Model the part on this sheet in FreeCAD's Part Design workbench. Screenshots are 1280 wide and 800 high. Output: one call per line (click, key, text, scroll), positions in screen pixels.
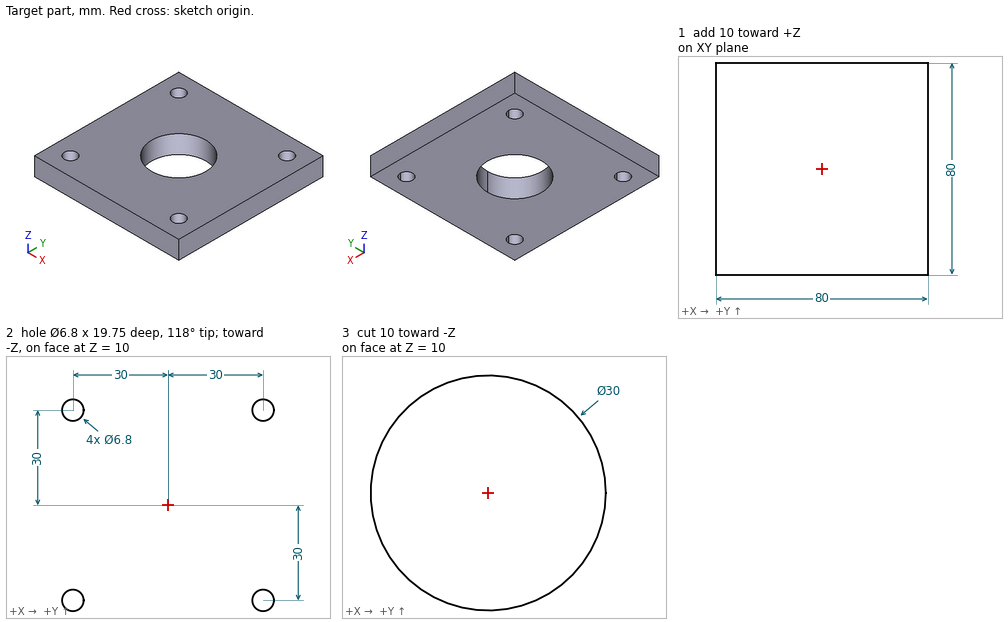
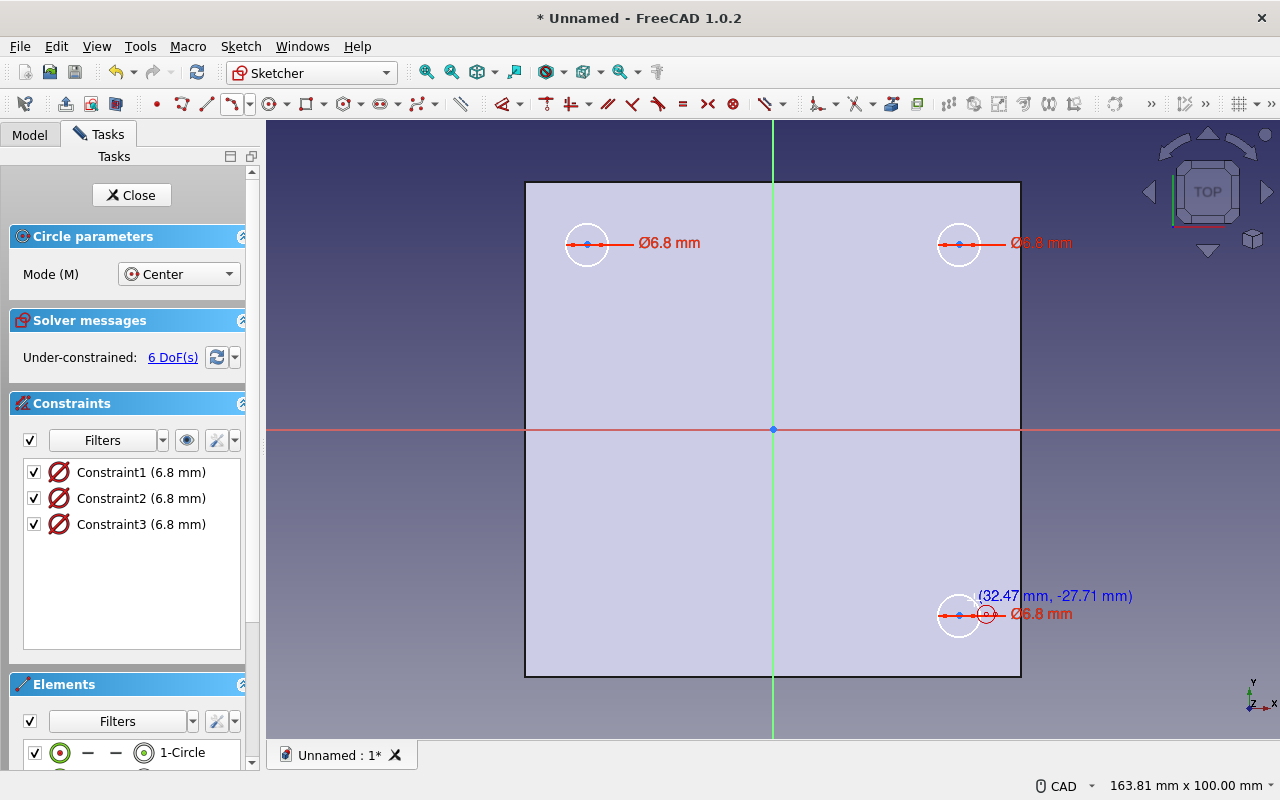
click(587, 615)
move(602, 600)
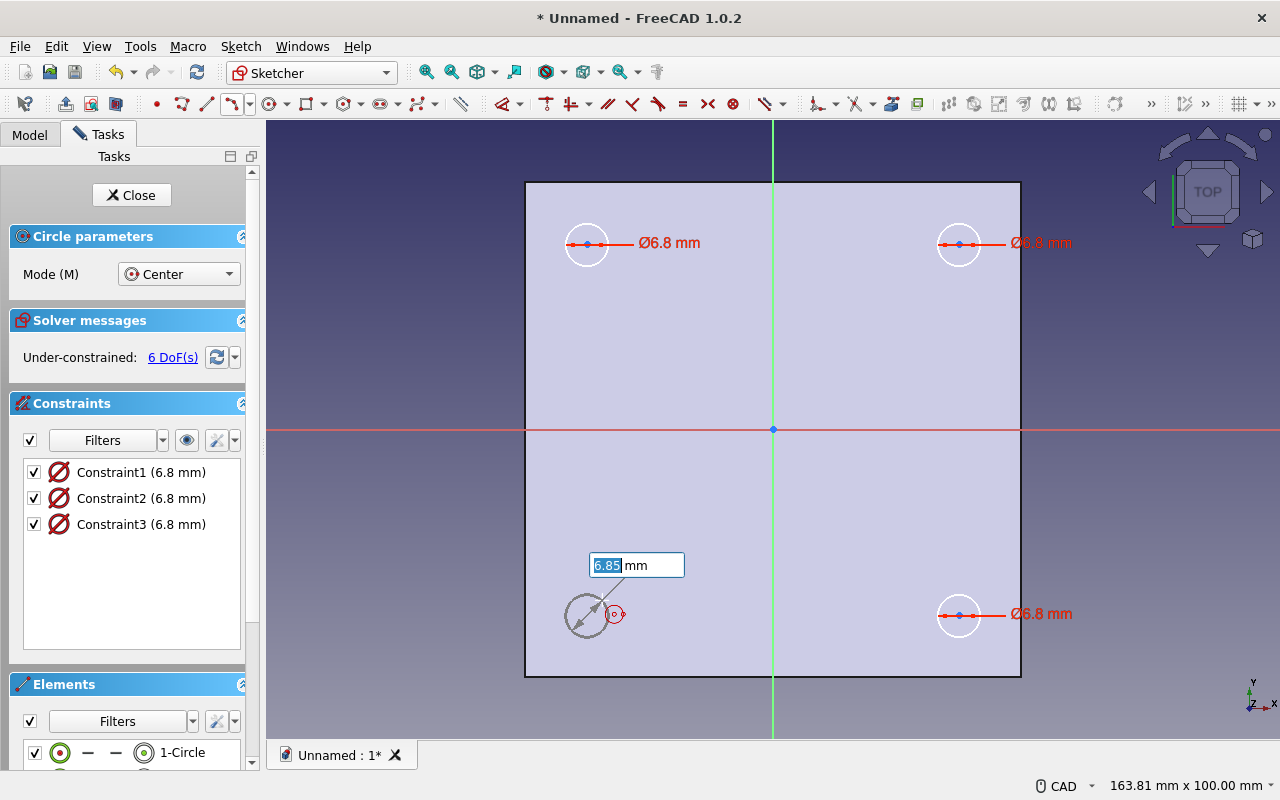
text(6.8)
key(Return)
key(Escape)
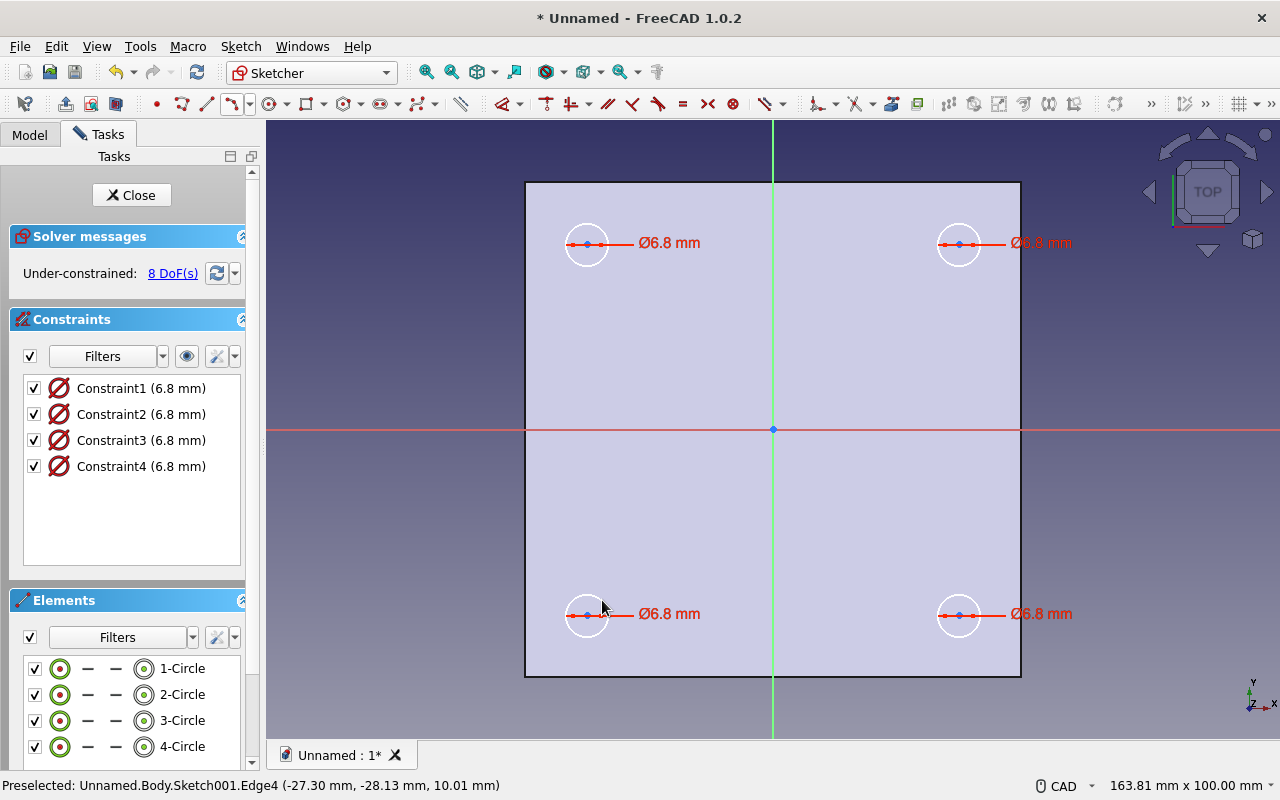
click(587, 245)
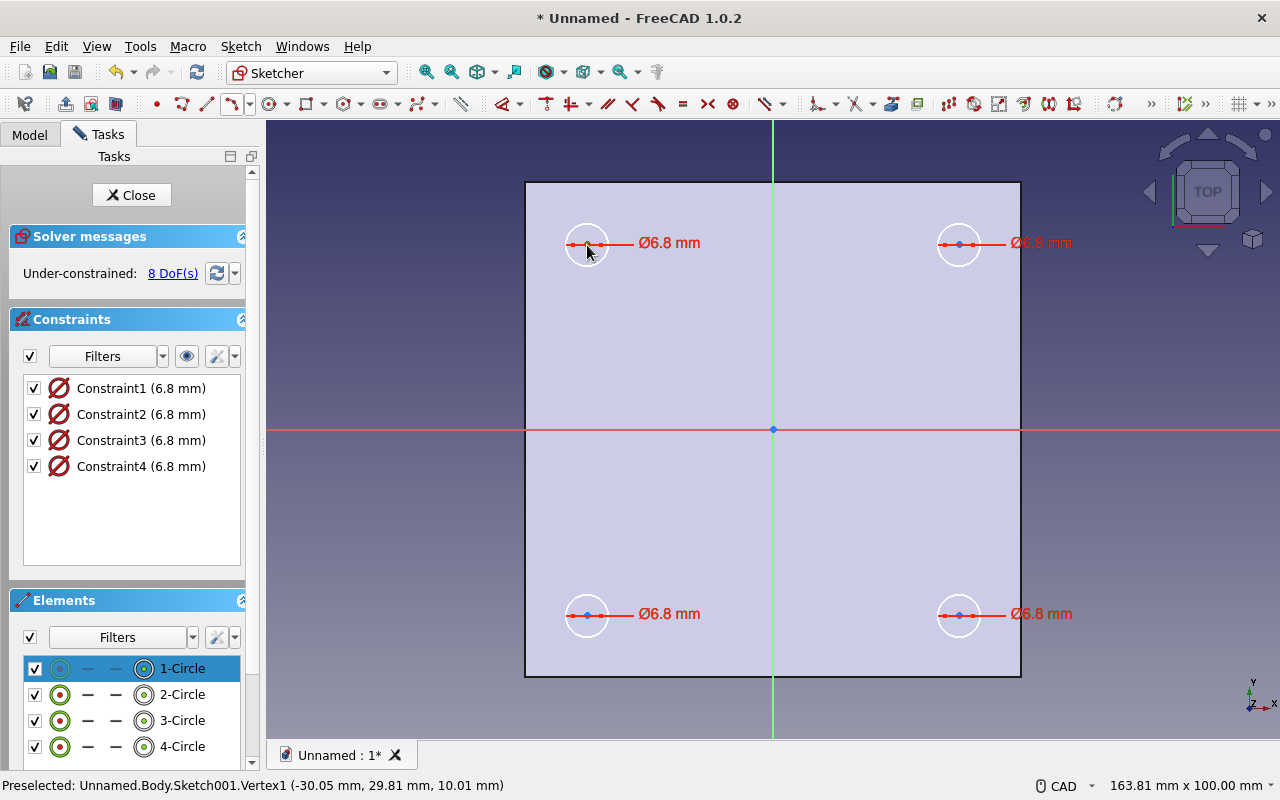
click(959, 245)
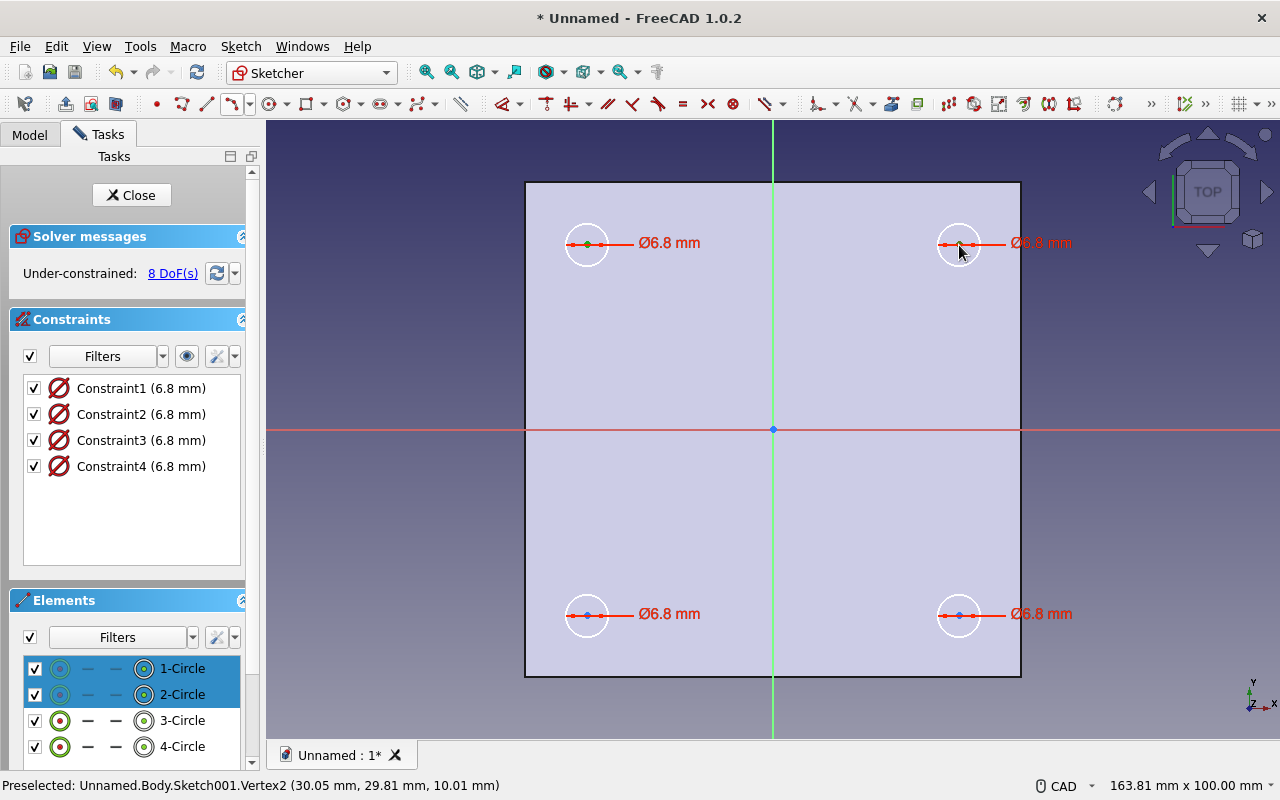
click(588, 104)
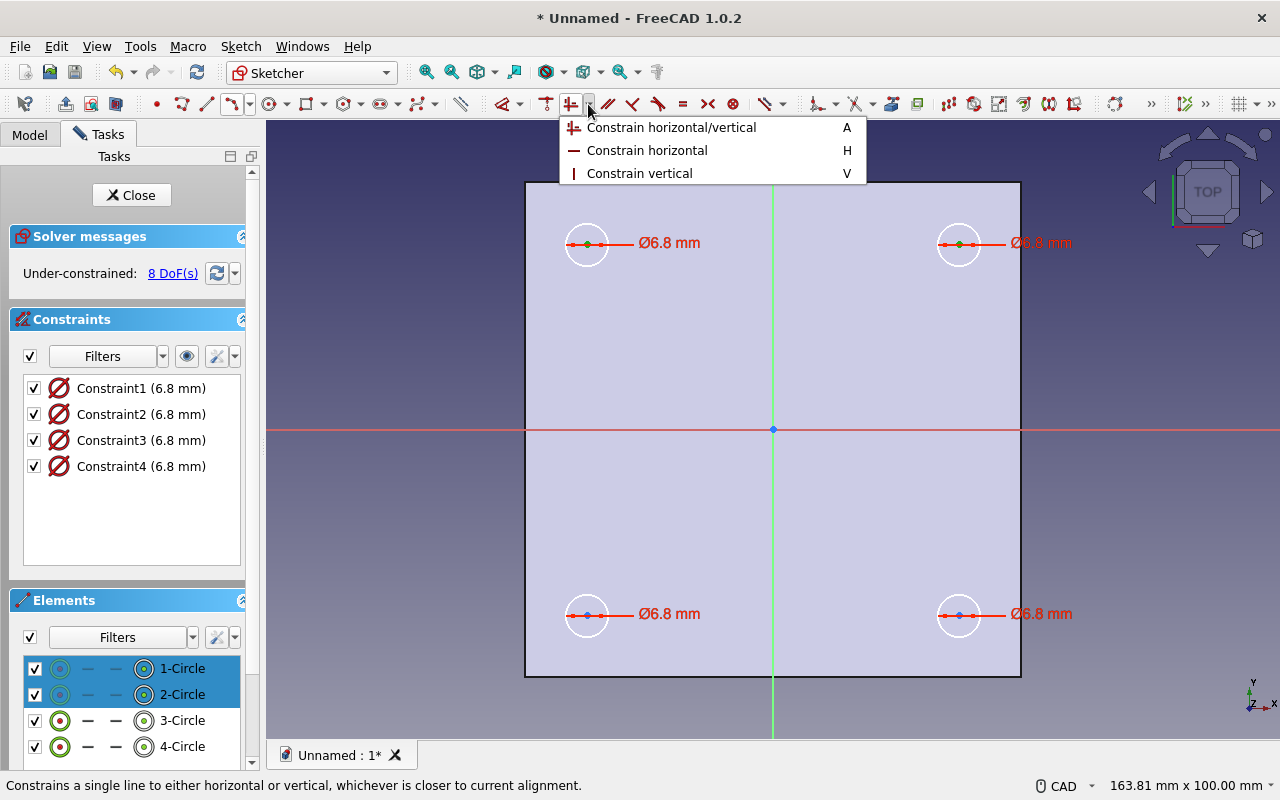
click(713, 150)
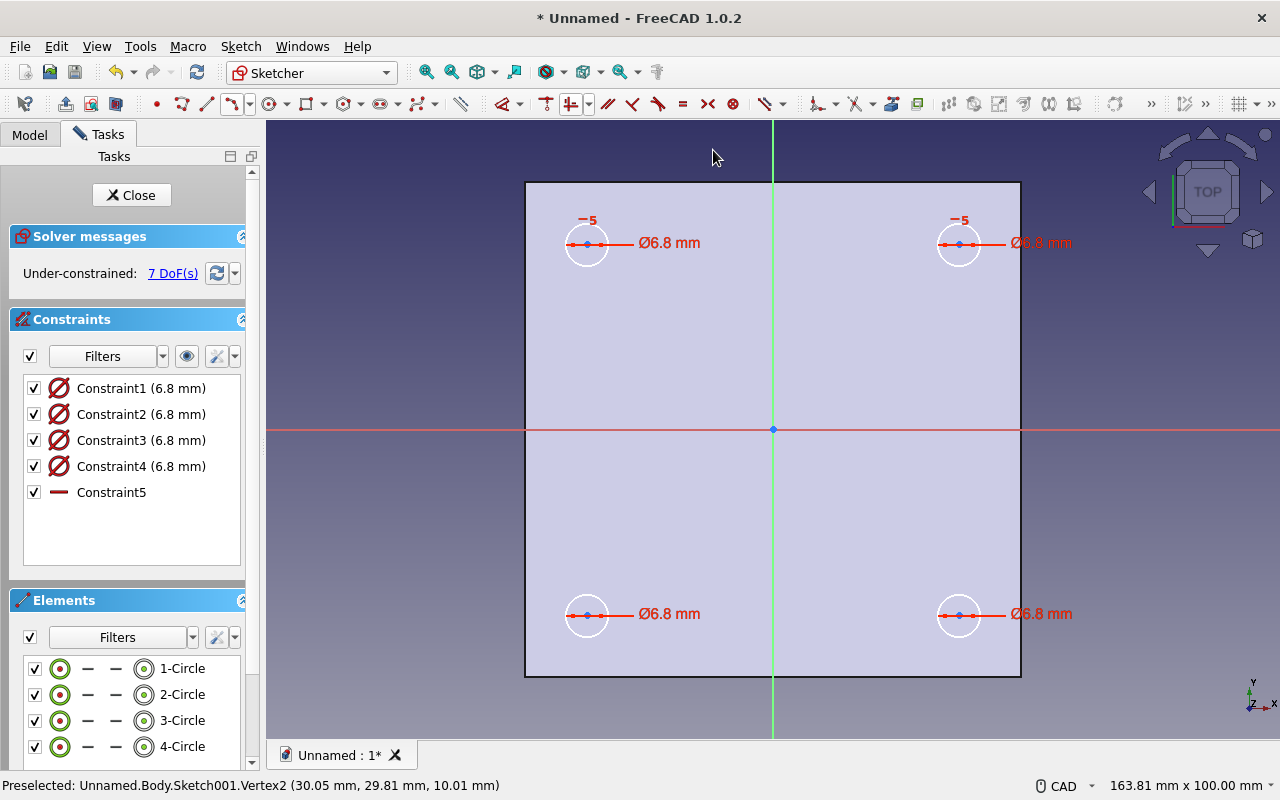
click(959, 245)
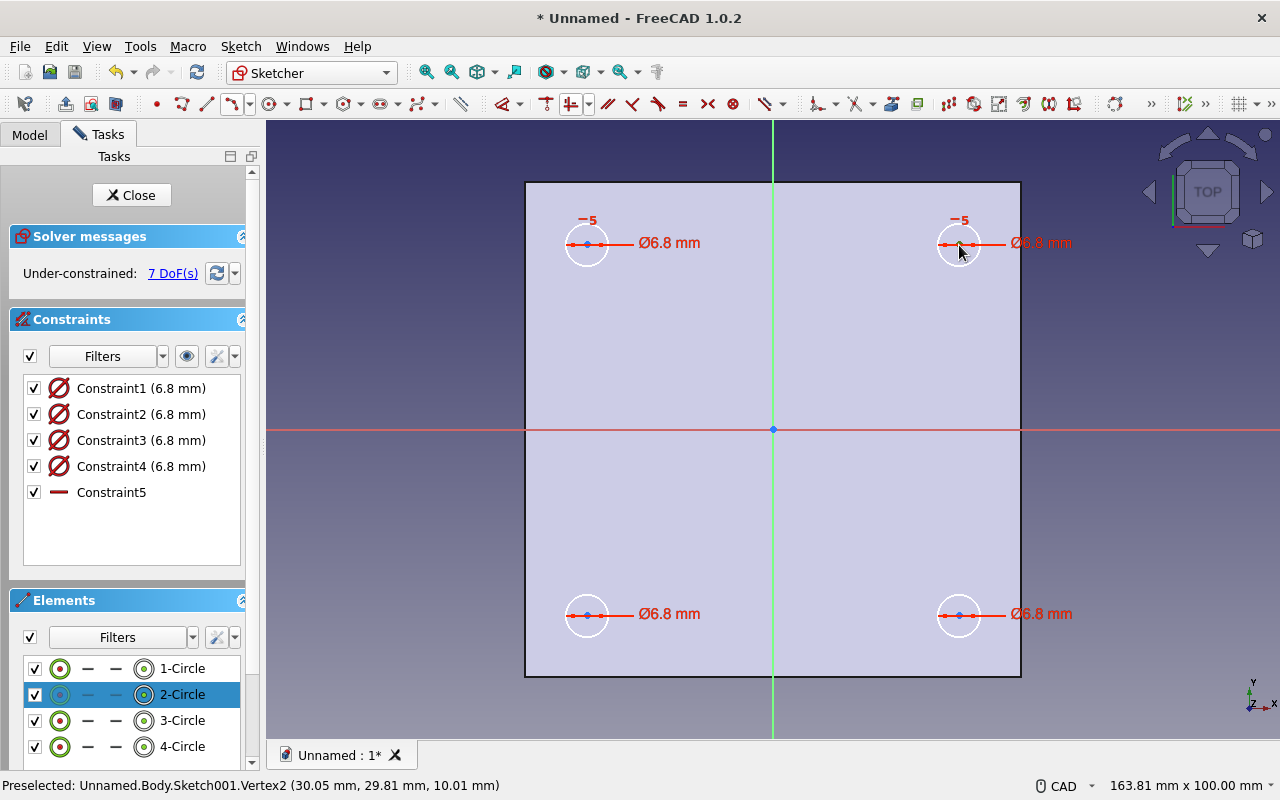
click(959, 616)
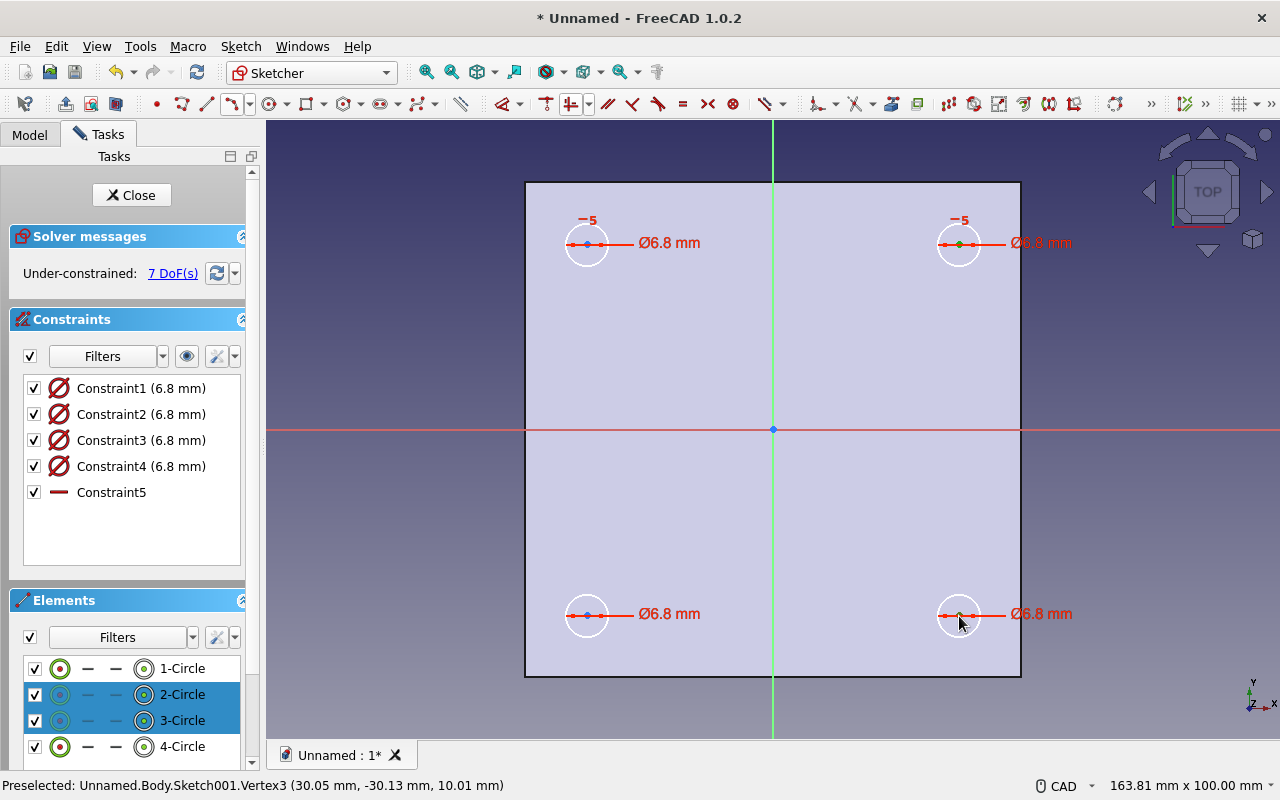
key(v)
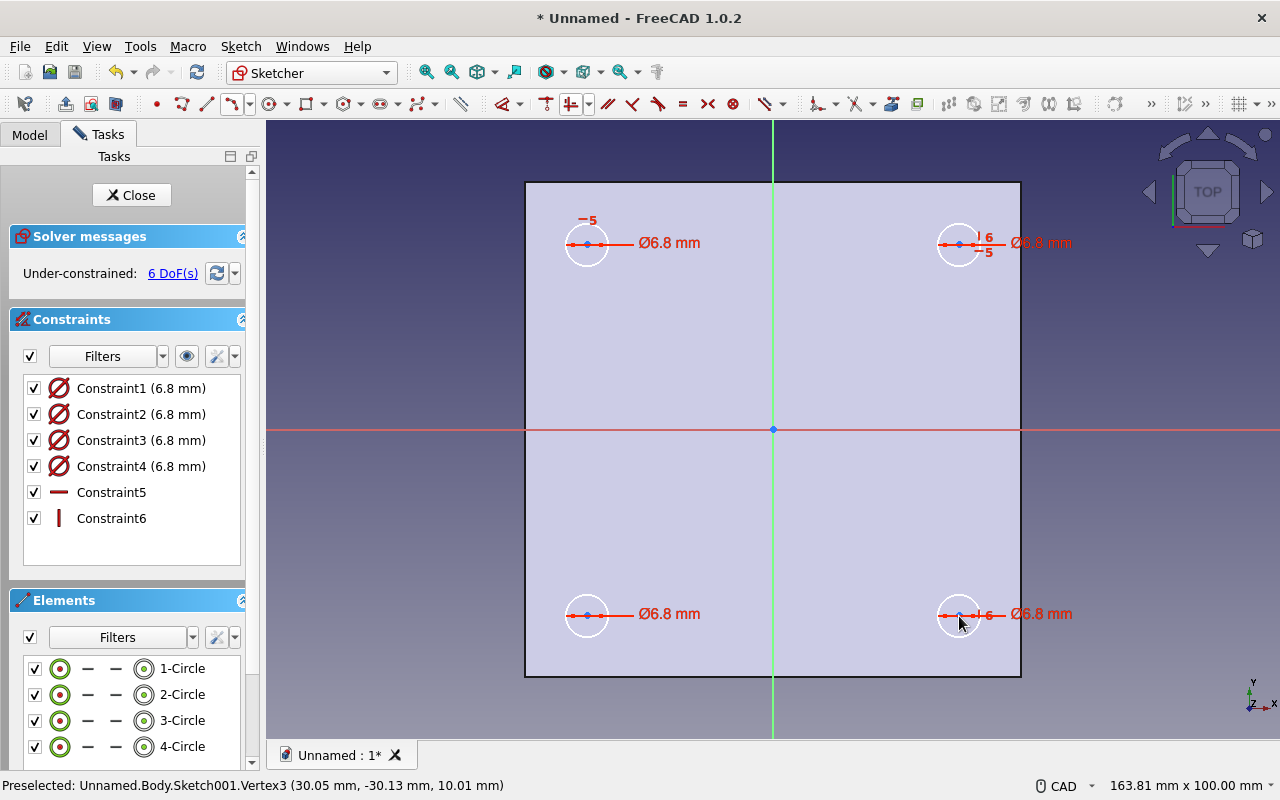
click(587, 245)